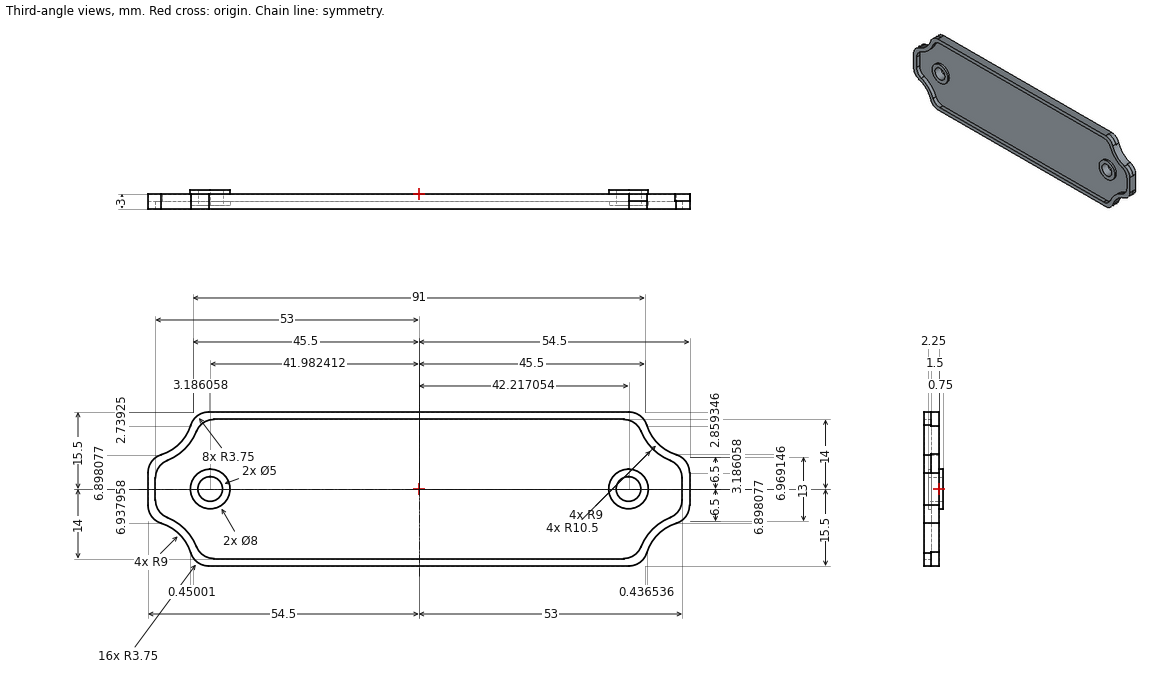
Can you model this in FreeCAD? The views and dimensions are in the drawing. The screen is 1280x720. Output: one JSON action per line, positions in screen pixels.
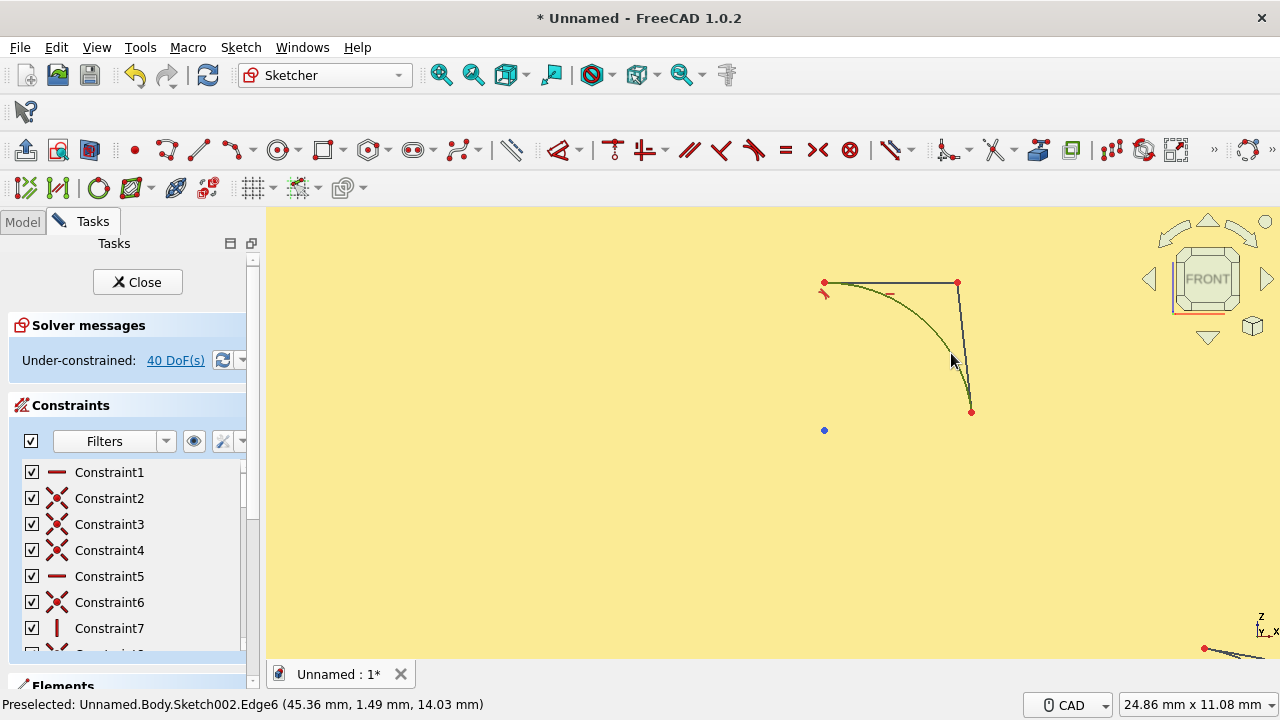
{"action": "scroll", "coordinate": [956, 356], "scroll_direction": "down", "scroll_amount": 10}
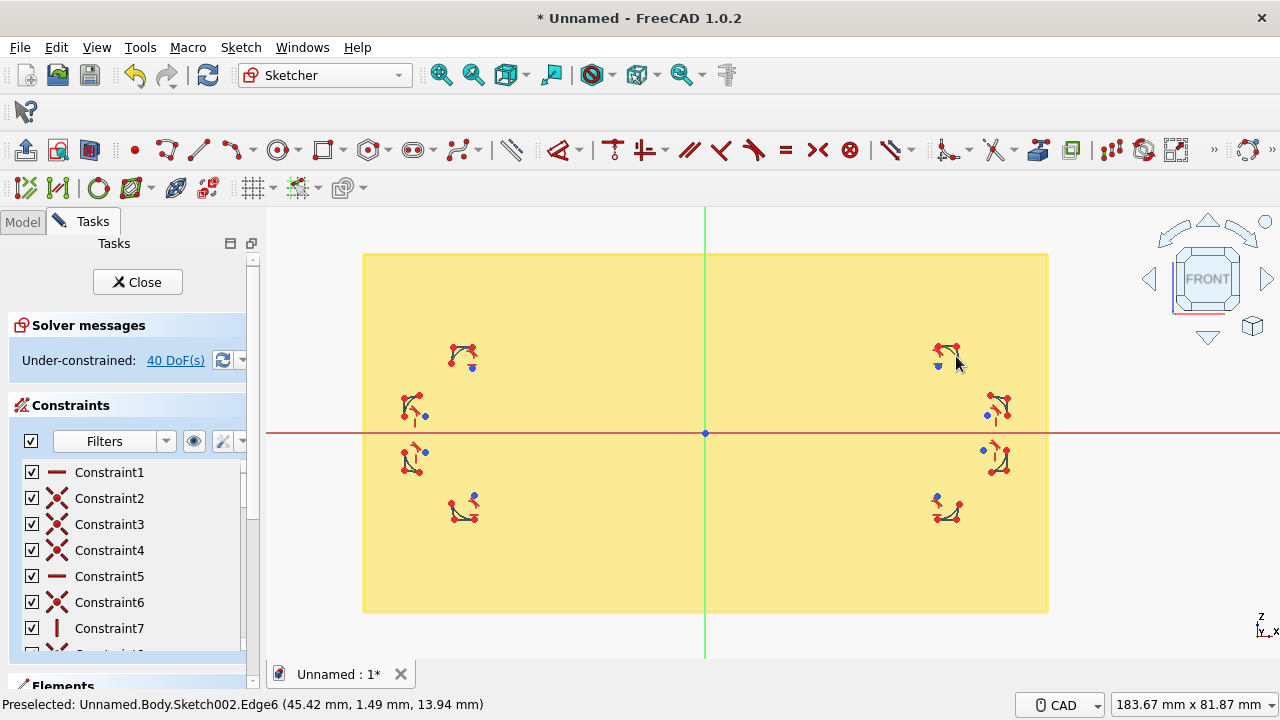
{"action": "scroll", "coordinate": [1006, 407], "scroll_direction": "up", "scroll_amount": 11}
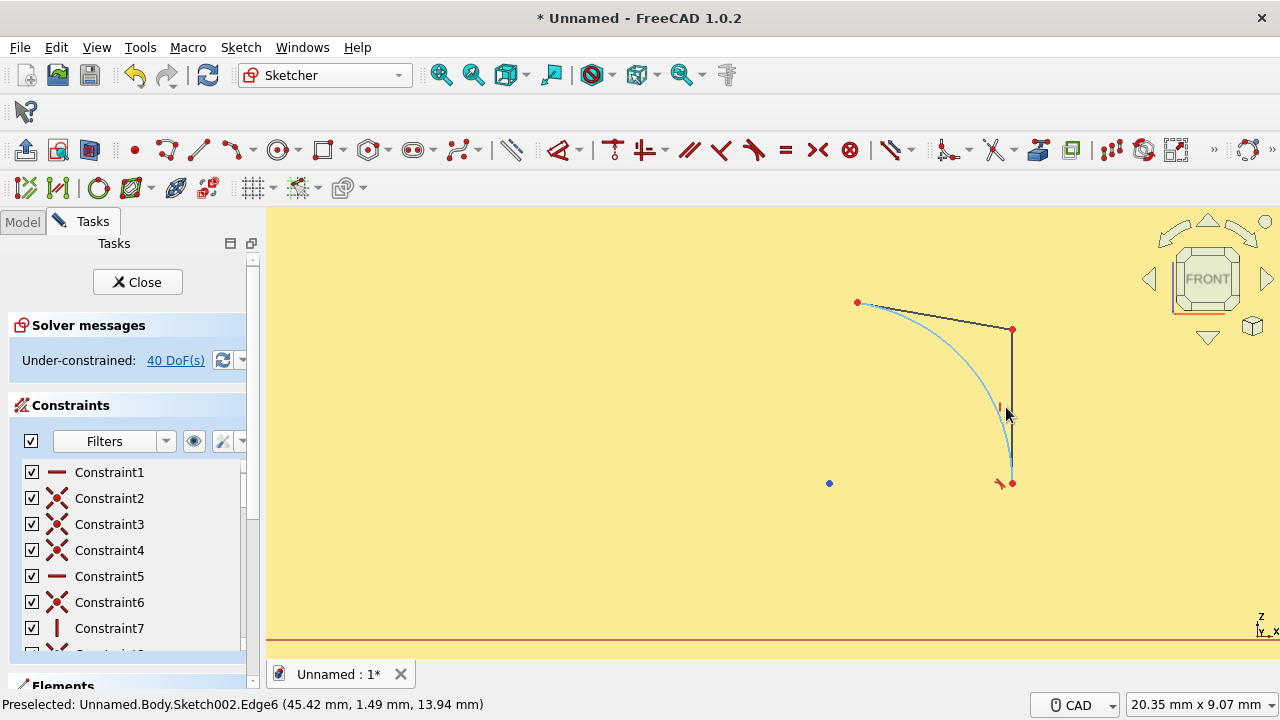
{"action": "left_click", "coordinate": [929, 330]}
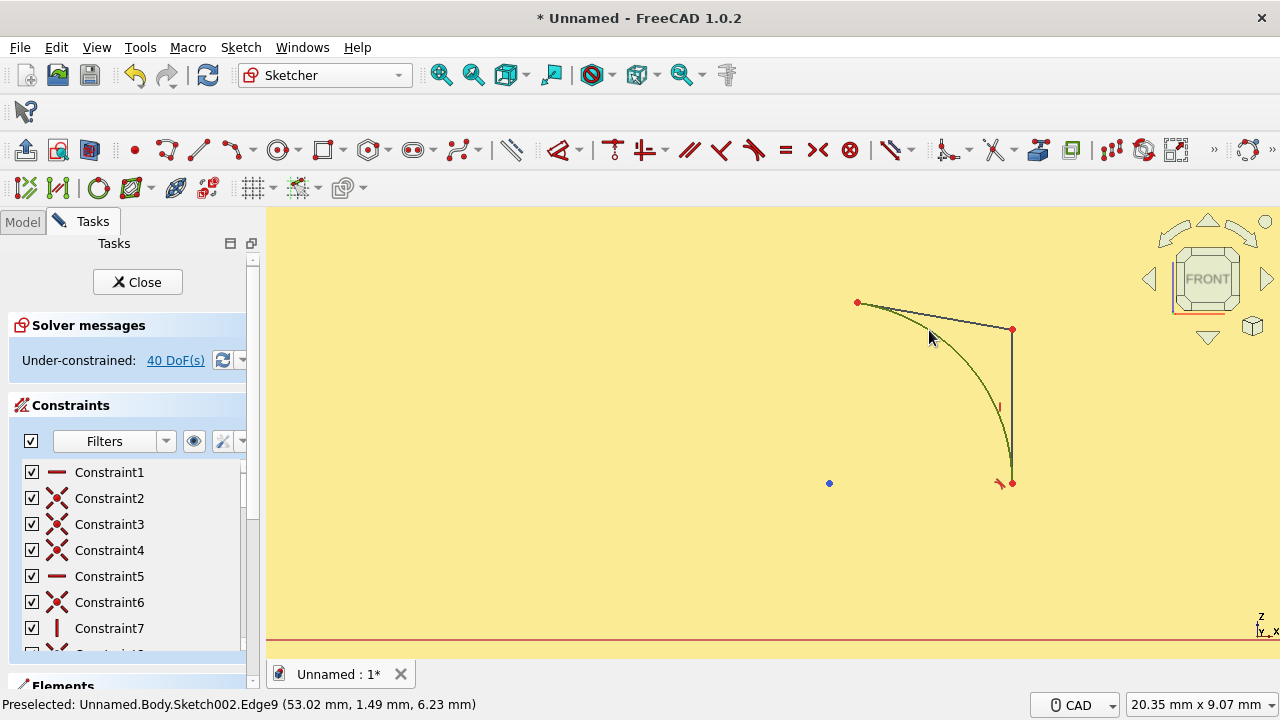
{"action": "scroll", "coordinate": [1006, 407], "scroll_direction": "down", "scroll_amount": 11}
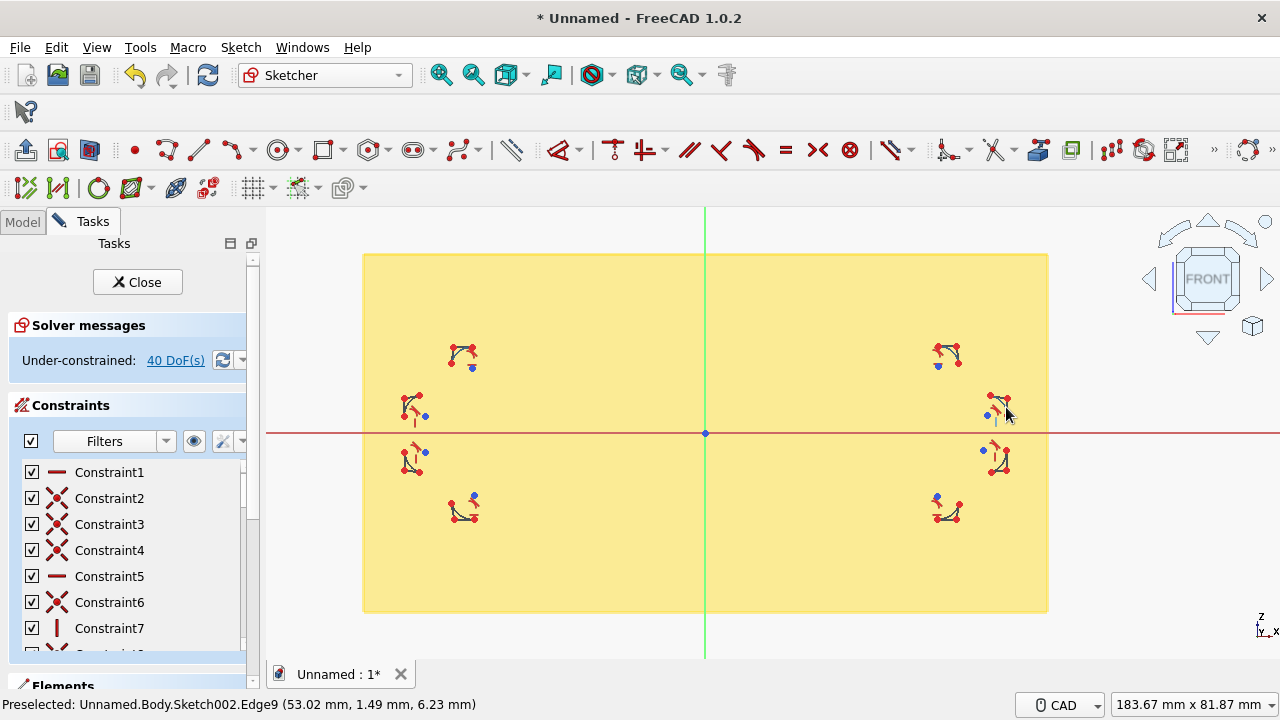
{"action": "scroll", "coordinate": [999, 468], "scroll_direction": "up", "scroll_amount": 8}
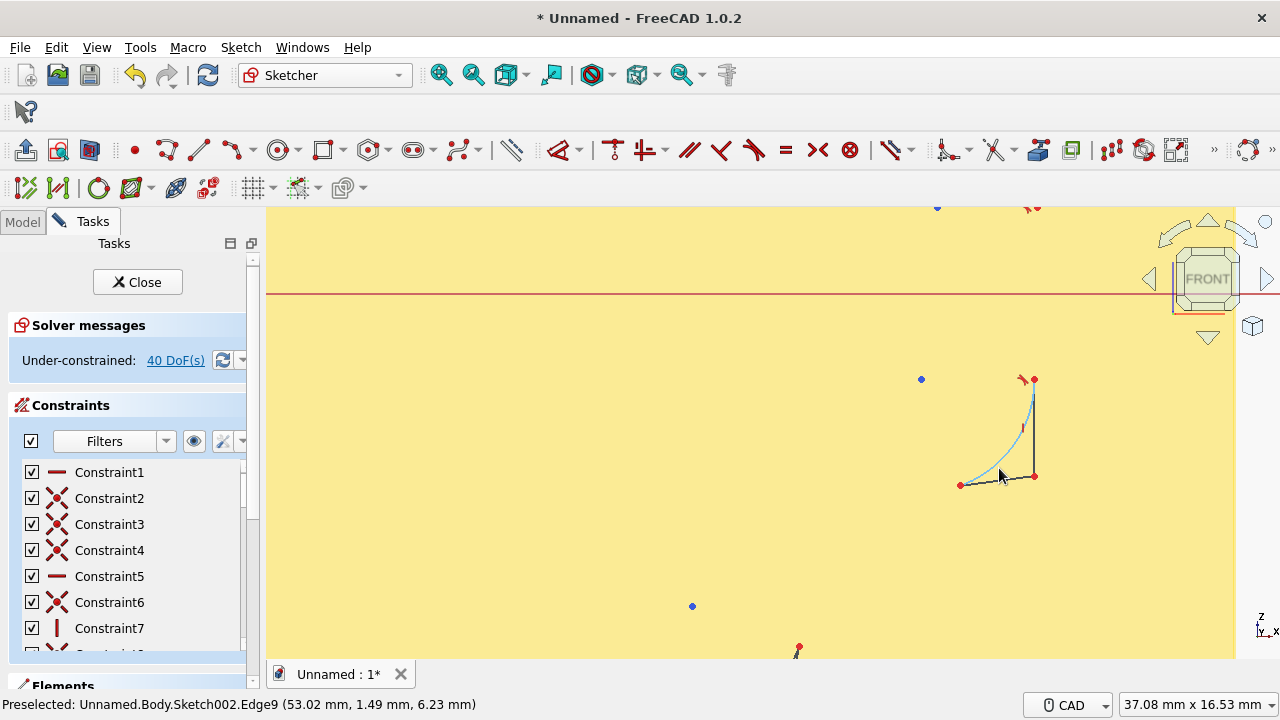
{"action": "left_click", "coordinate": [996, 465]}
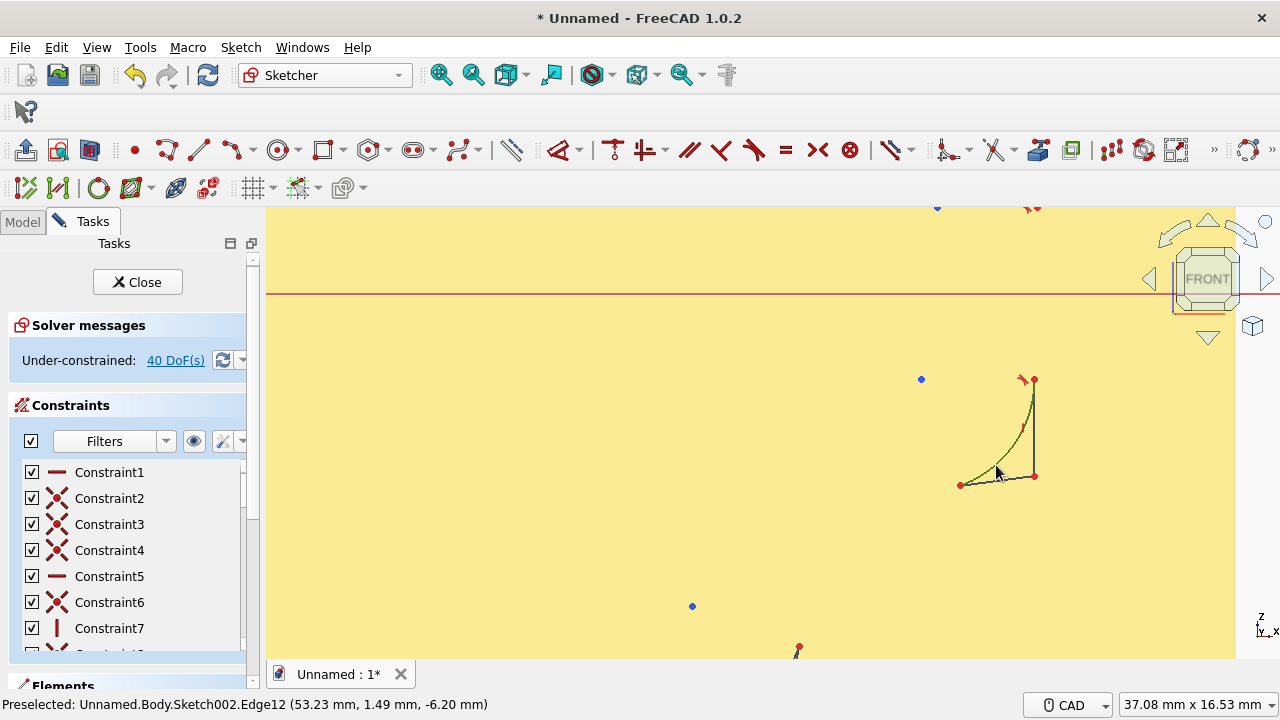
{"action": "scroll", "coordinate": [999, 468], "scroll_direction": "down", "scroll_amount": 8}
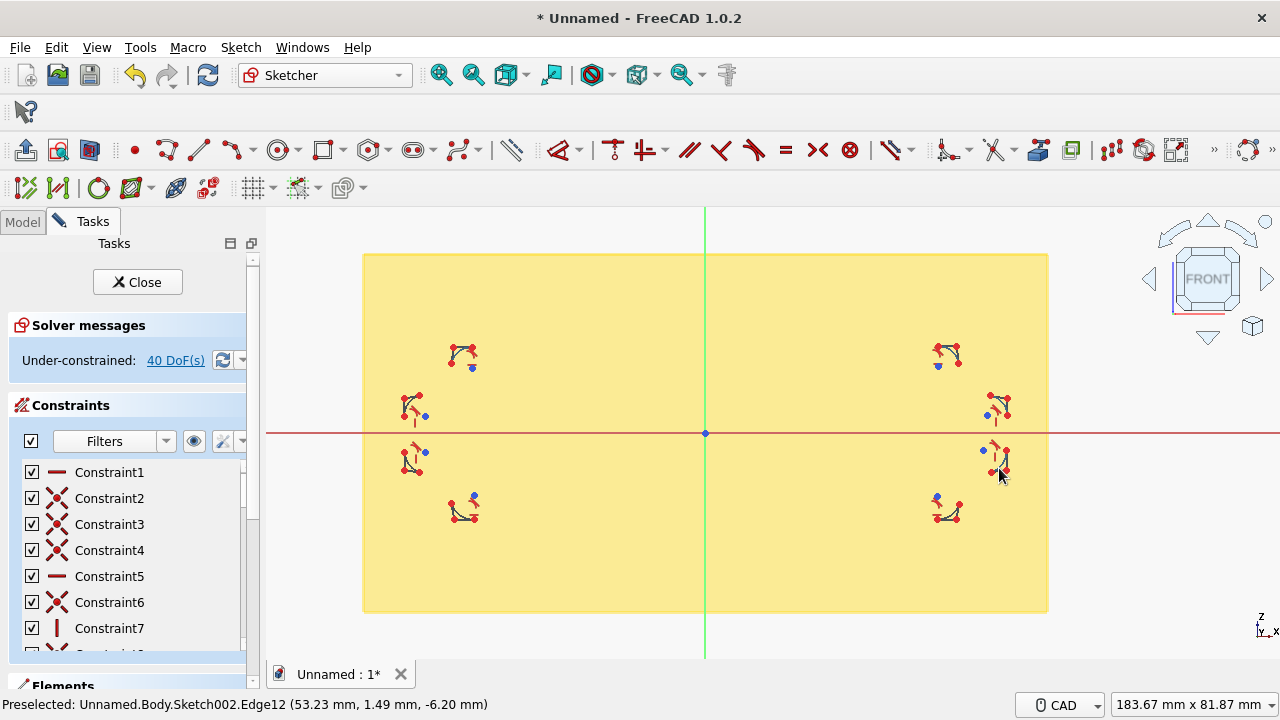
{"action": "scroll", "coordinate": [955, 512], "scroll_direction": "up", "scroll_amount": 9}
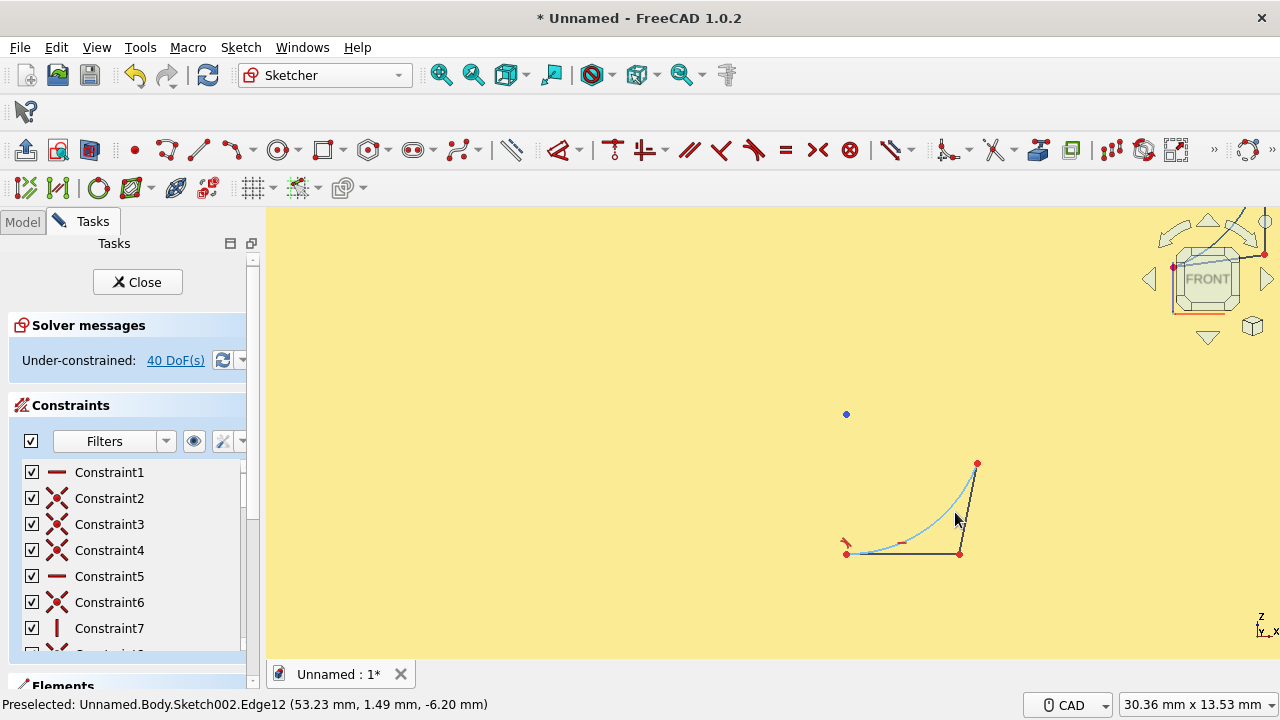
{"action": "left_click", "coordinate": [951, 507]}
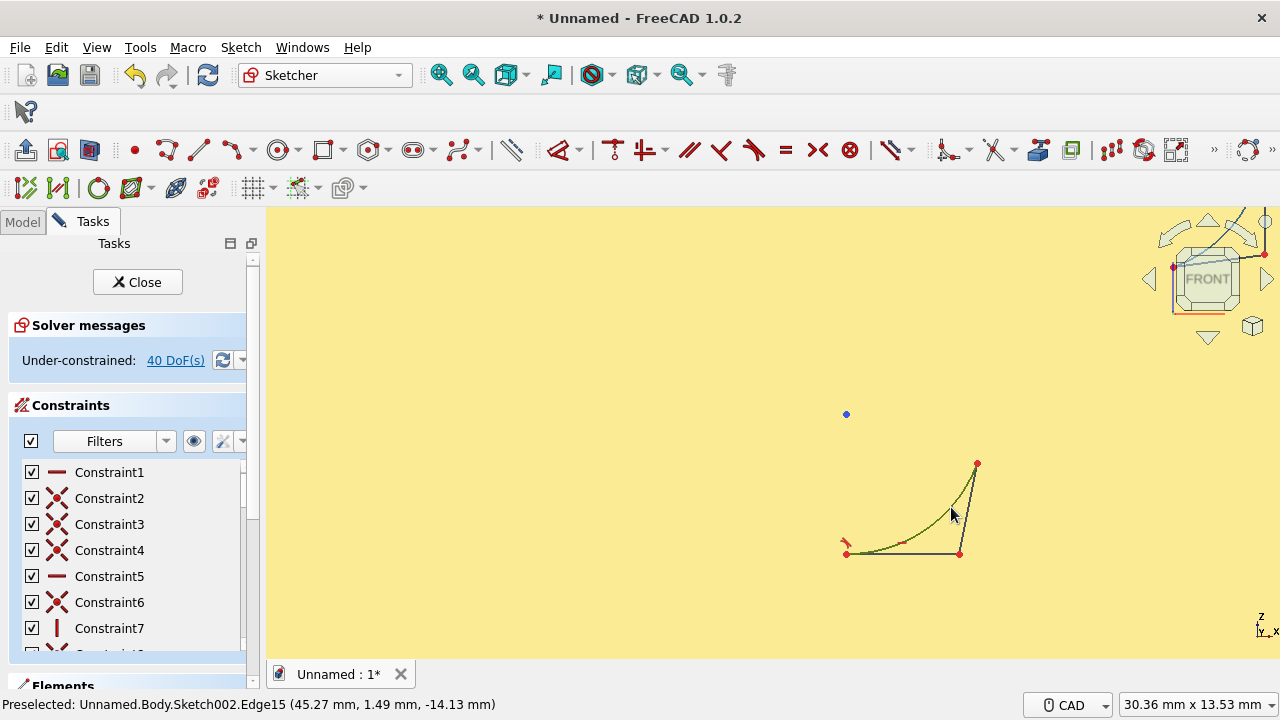
{"action": "scroll", "coordinate": [955, 512], "scroll_direction": "down", "scroll_amount": 9}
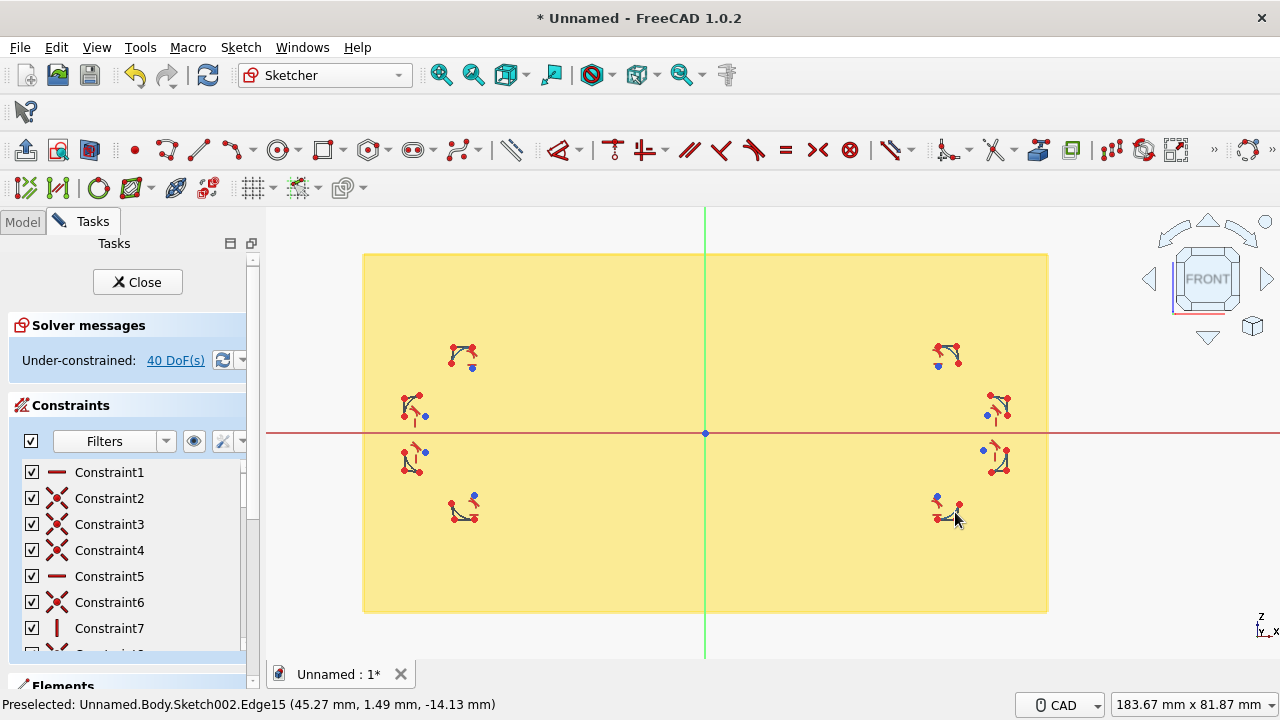
{"action": "scroll", "coordinate": [456, 512], "scroll_direction": "up", "scroll_amount": 8}